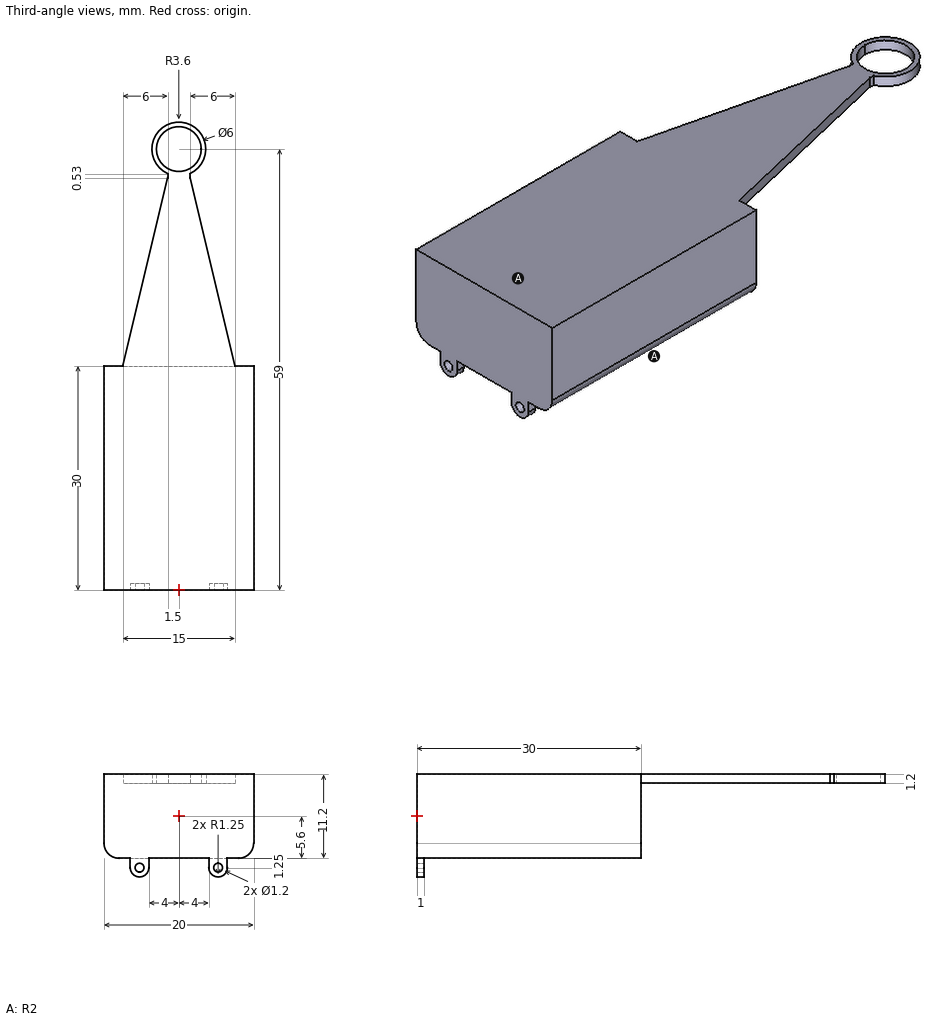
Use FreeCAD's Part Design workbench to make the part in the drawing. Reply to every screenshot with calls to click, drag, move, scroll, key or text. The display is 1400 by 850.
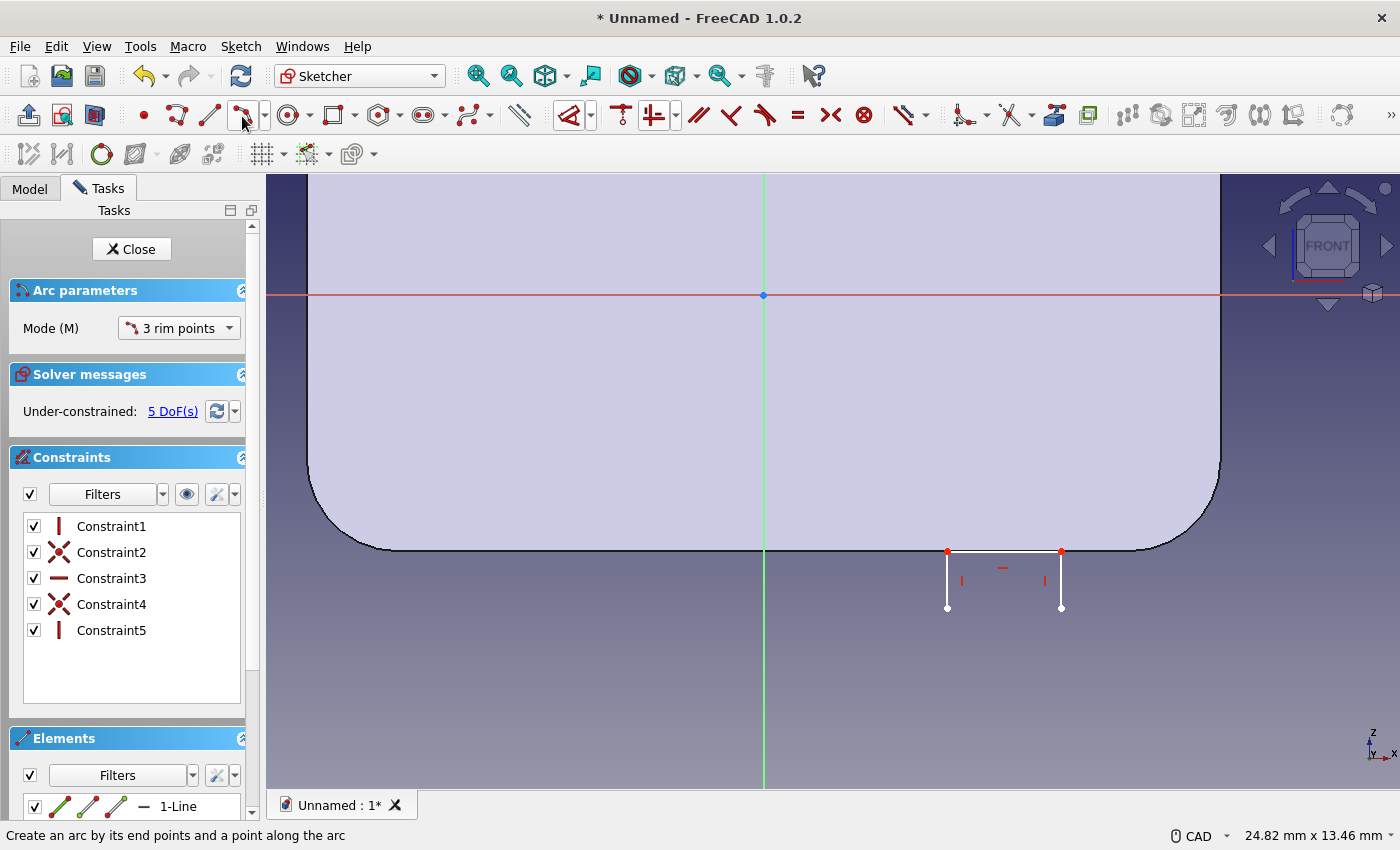
click(947, 609)
click(1061, 609)
click(1004, 666)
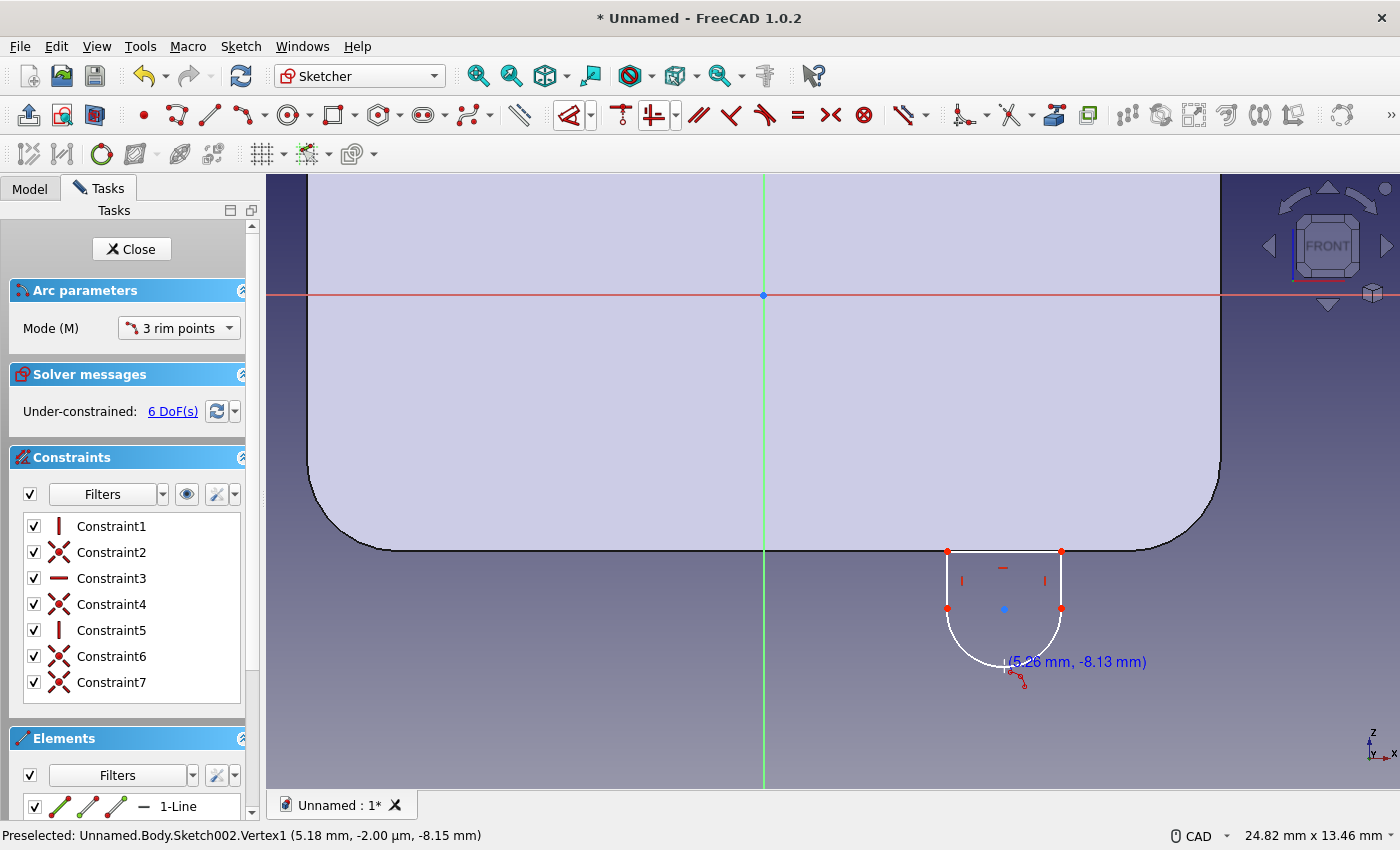
key(g)
key(m)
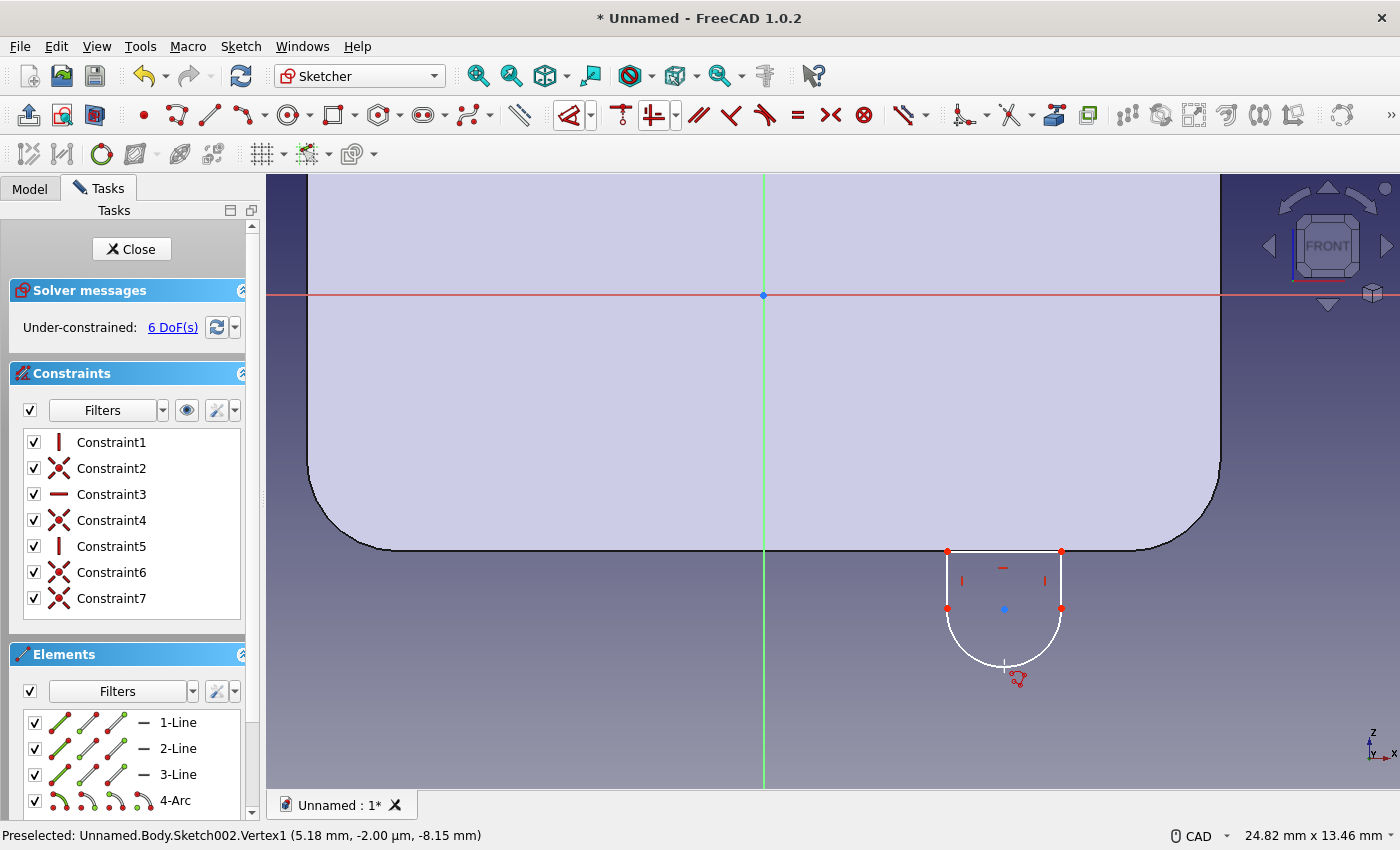
click(581, 608)
click(581, 551)
click(467, 551)
click(467, 608)
right_click(467, 608)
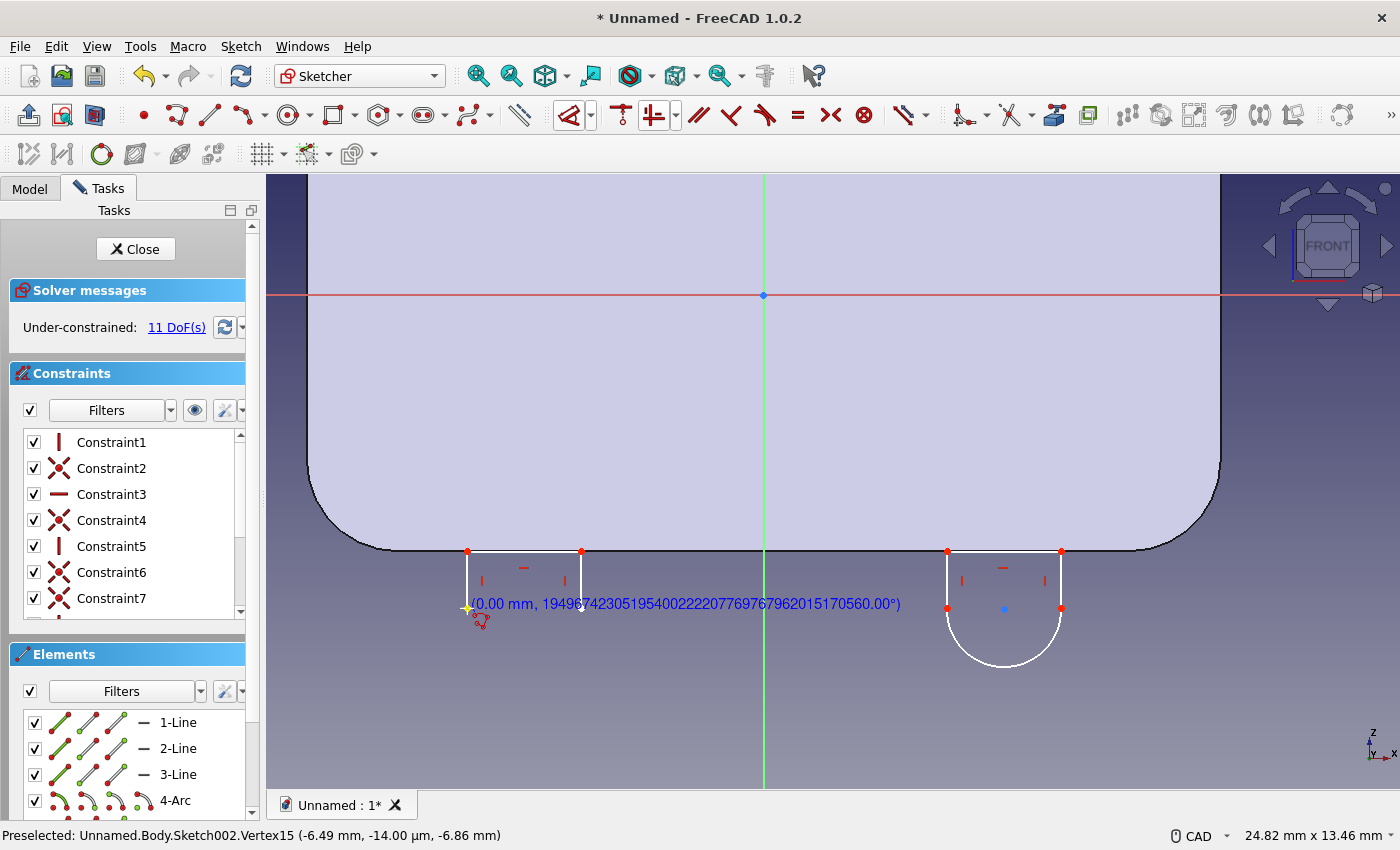
click(242, 116)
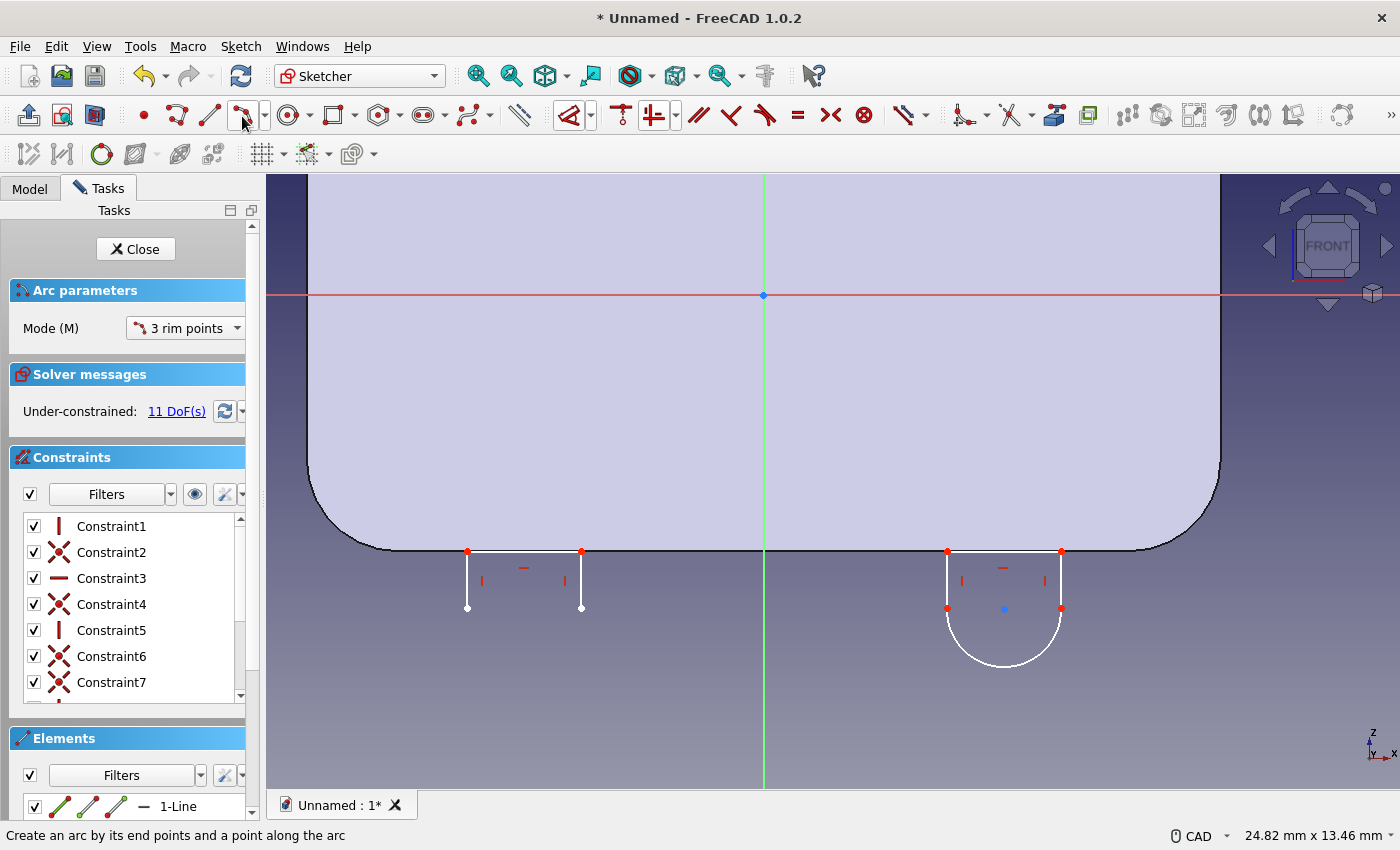
click(467, 609)
click(581, 609)
click(524, 666)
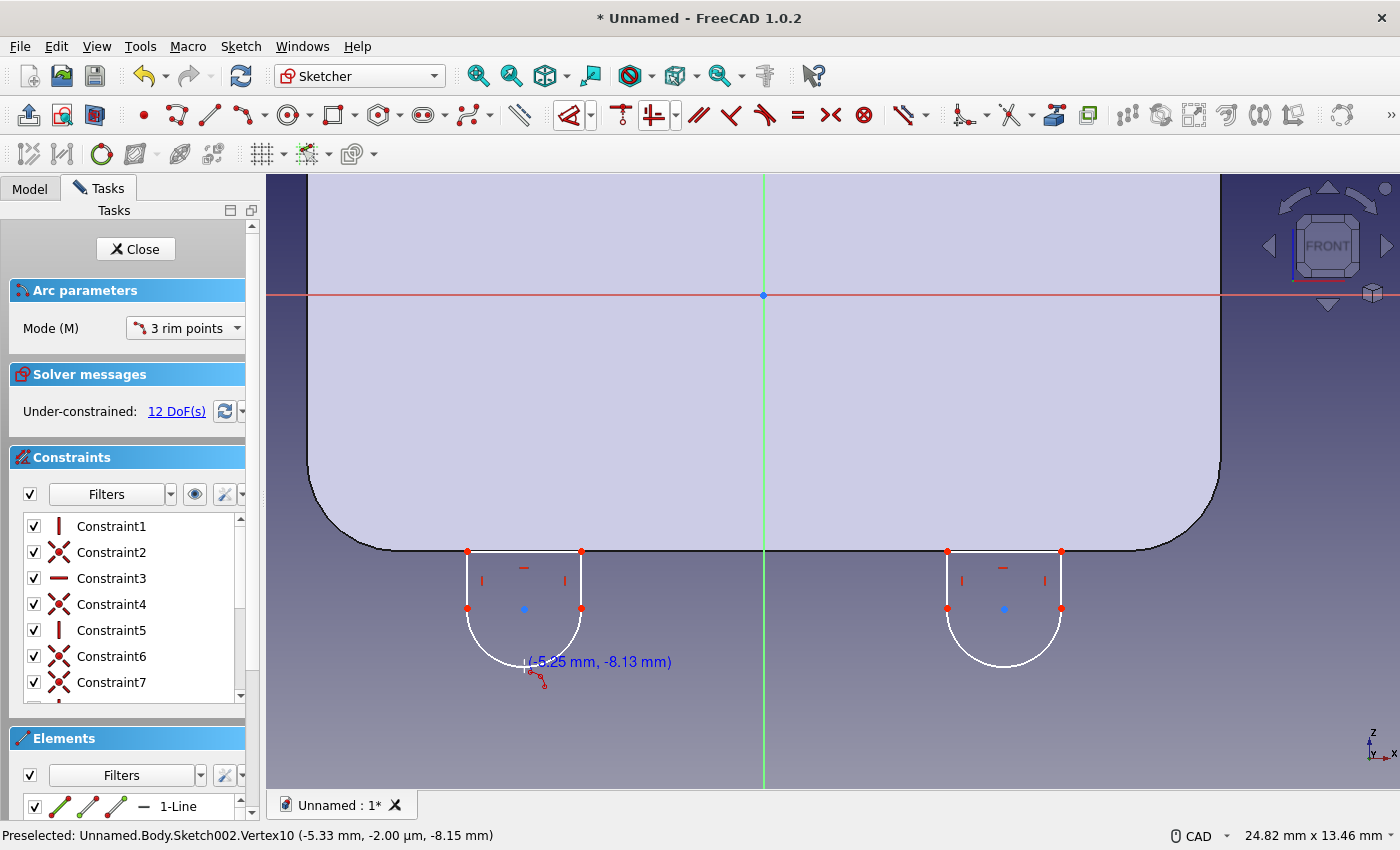
key(g)
key(c)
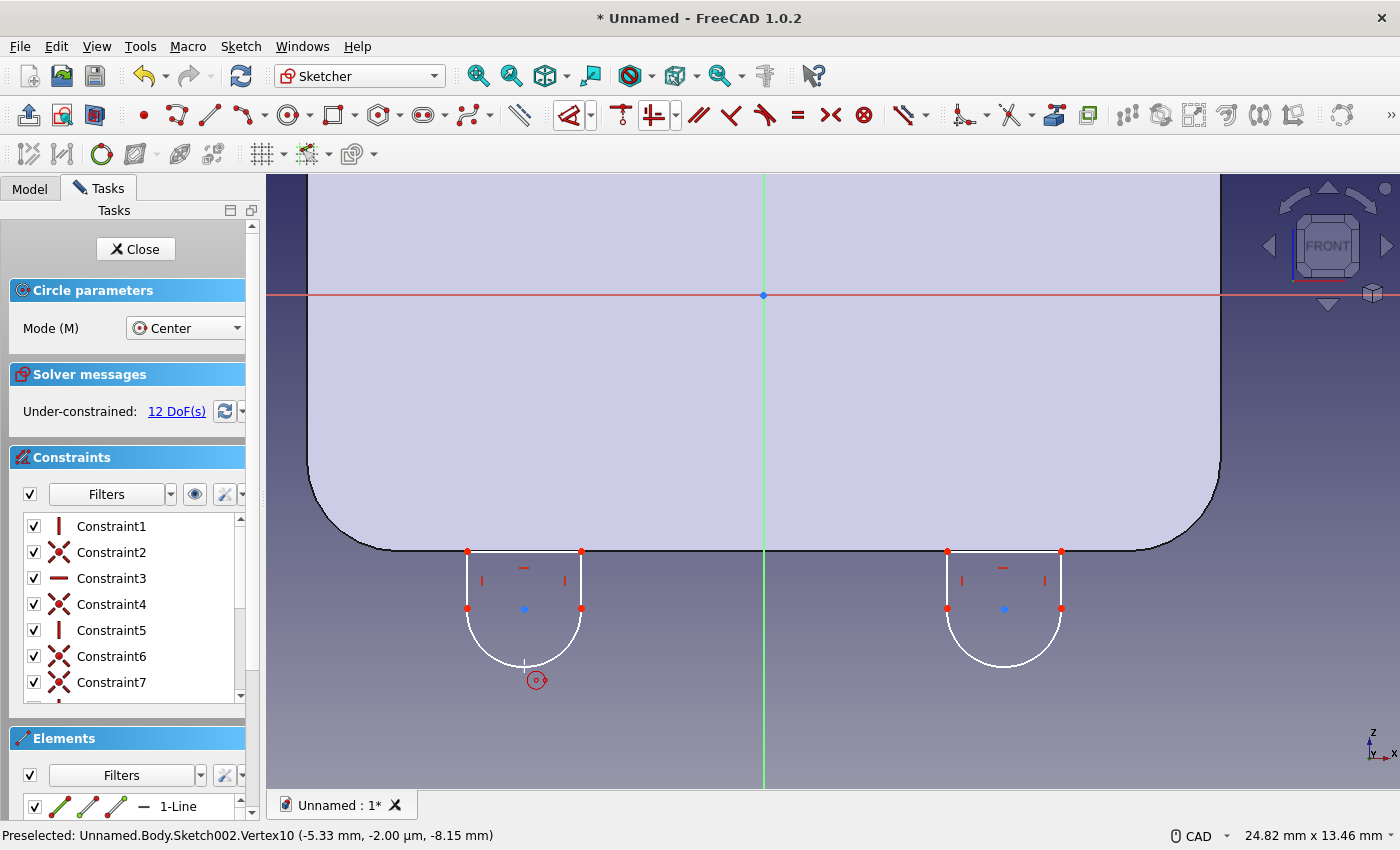
click(1004, 608)
click(1023, 589)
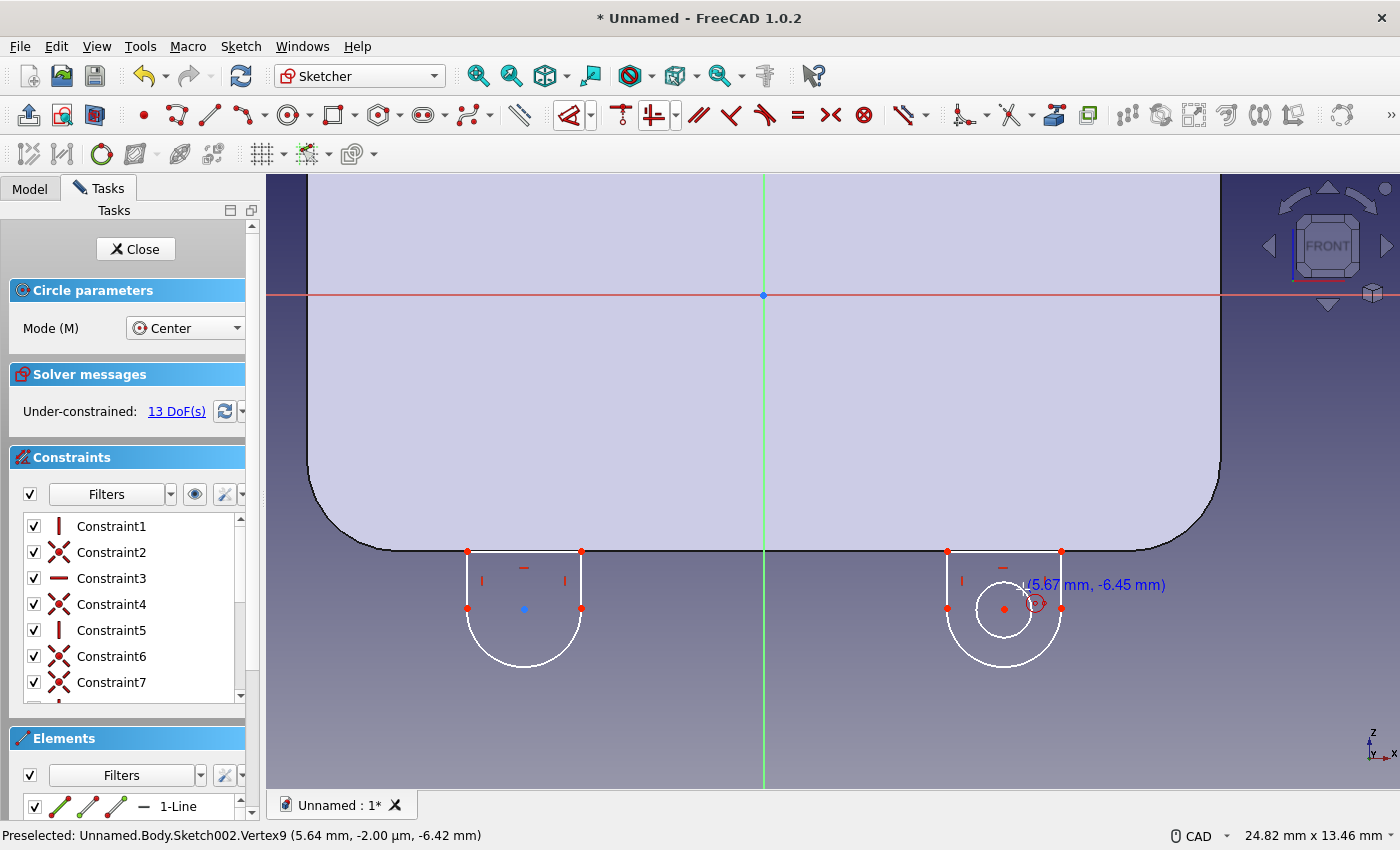
click(524, 608)
click(543, 589)
key(Escape)